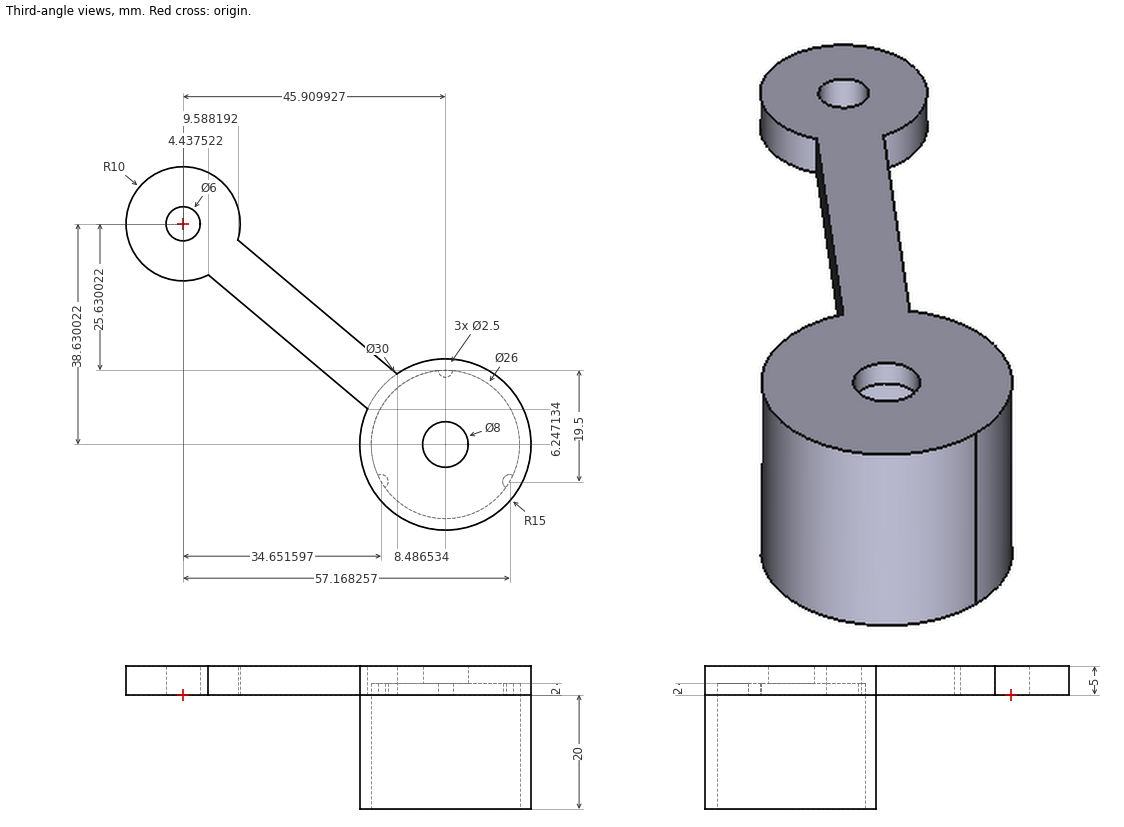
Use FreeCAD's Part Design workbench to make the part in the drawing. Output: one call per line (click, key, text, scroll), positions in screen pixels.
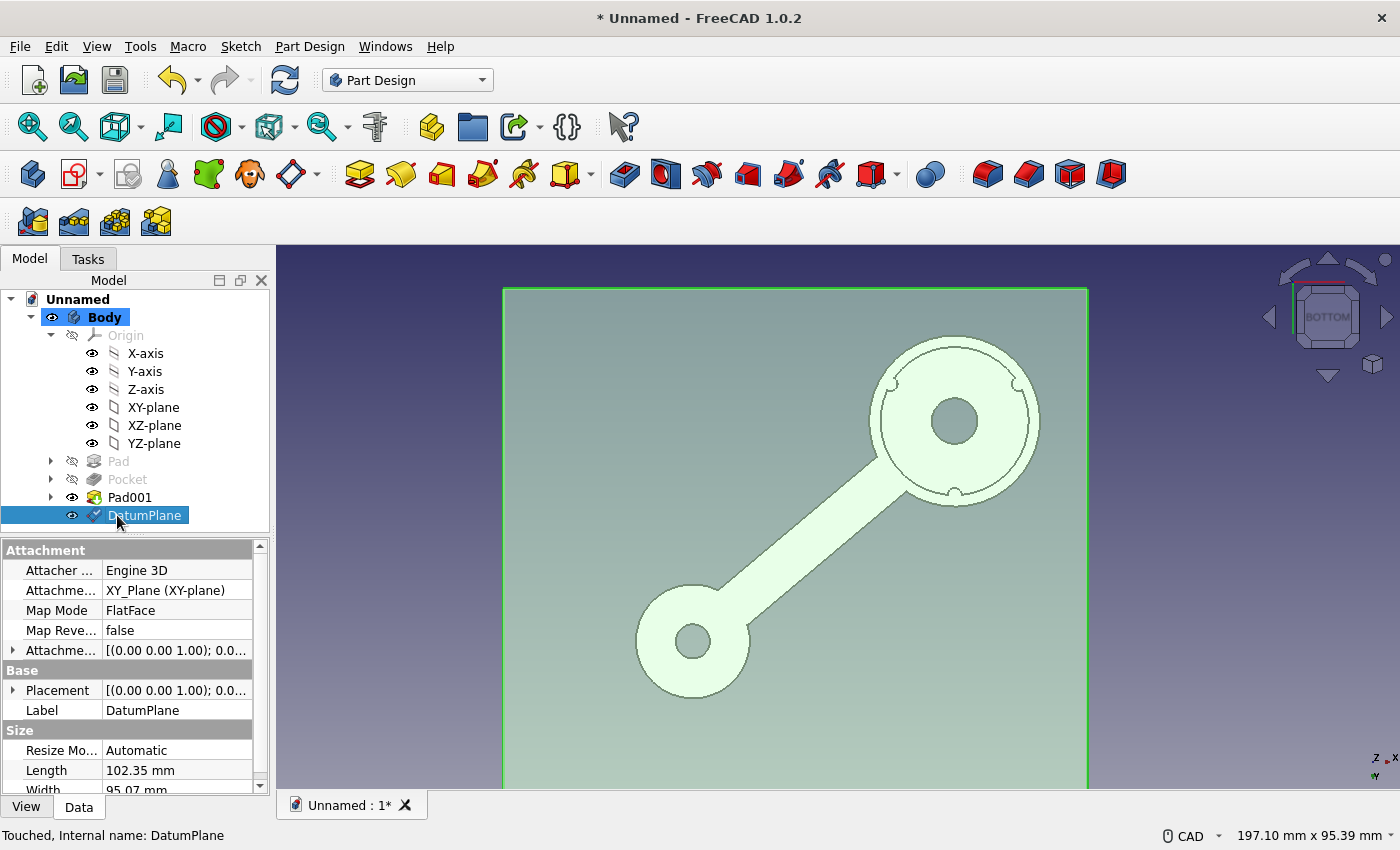
click(74, 174)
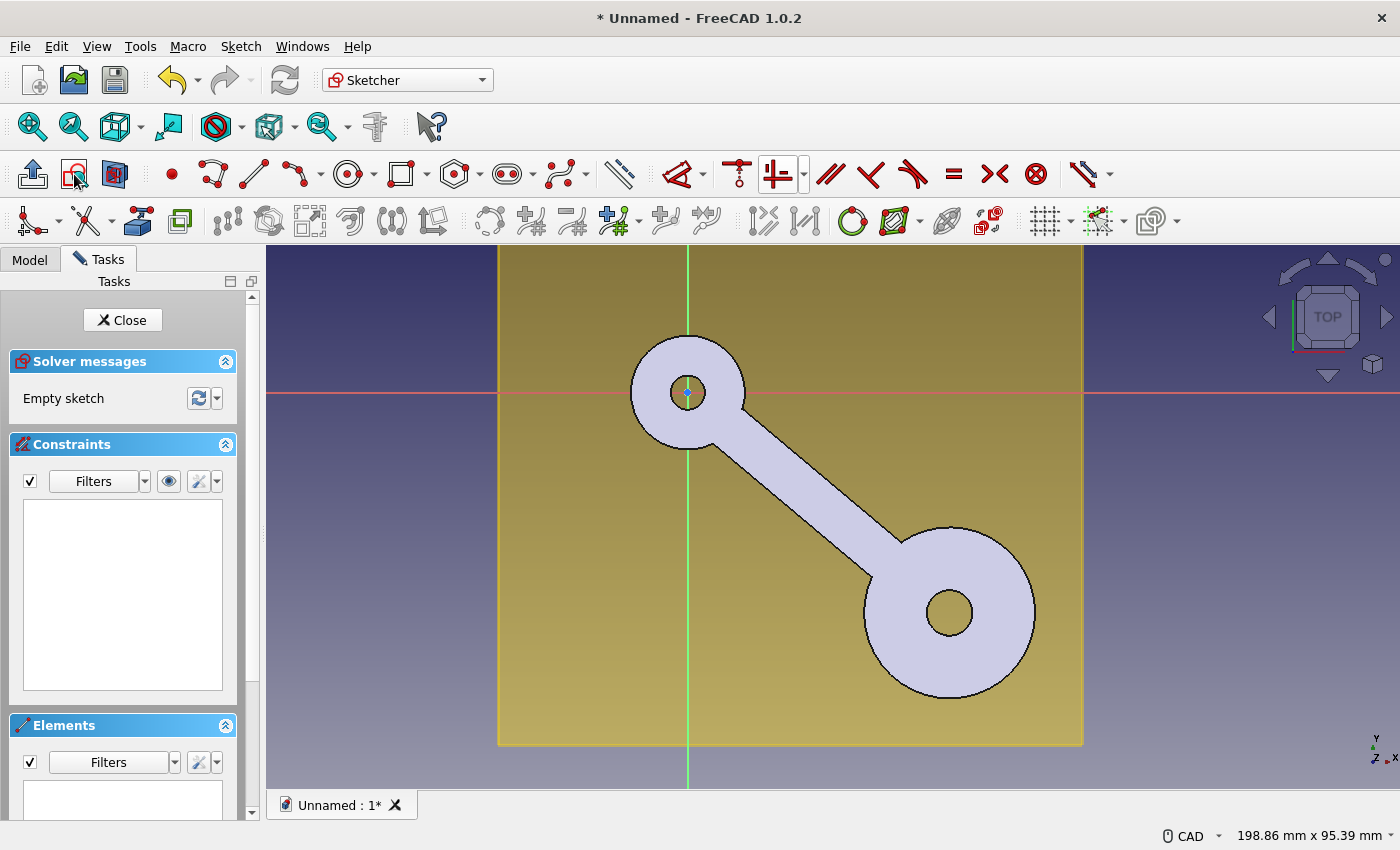
key(q)
key(s)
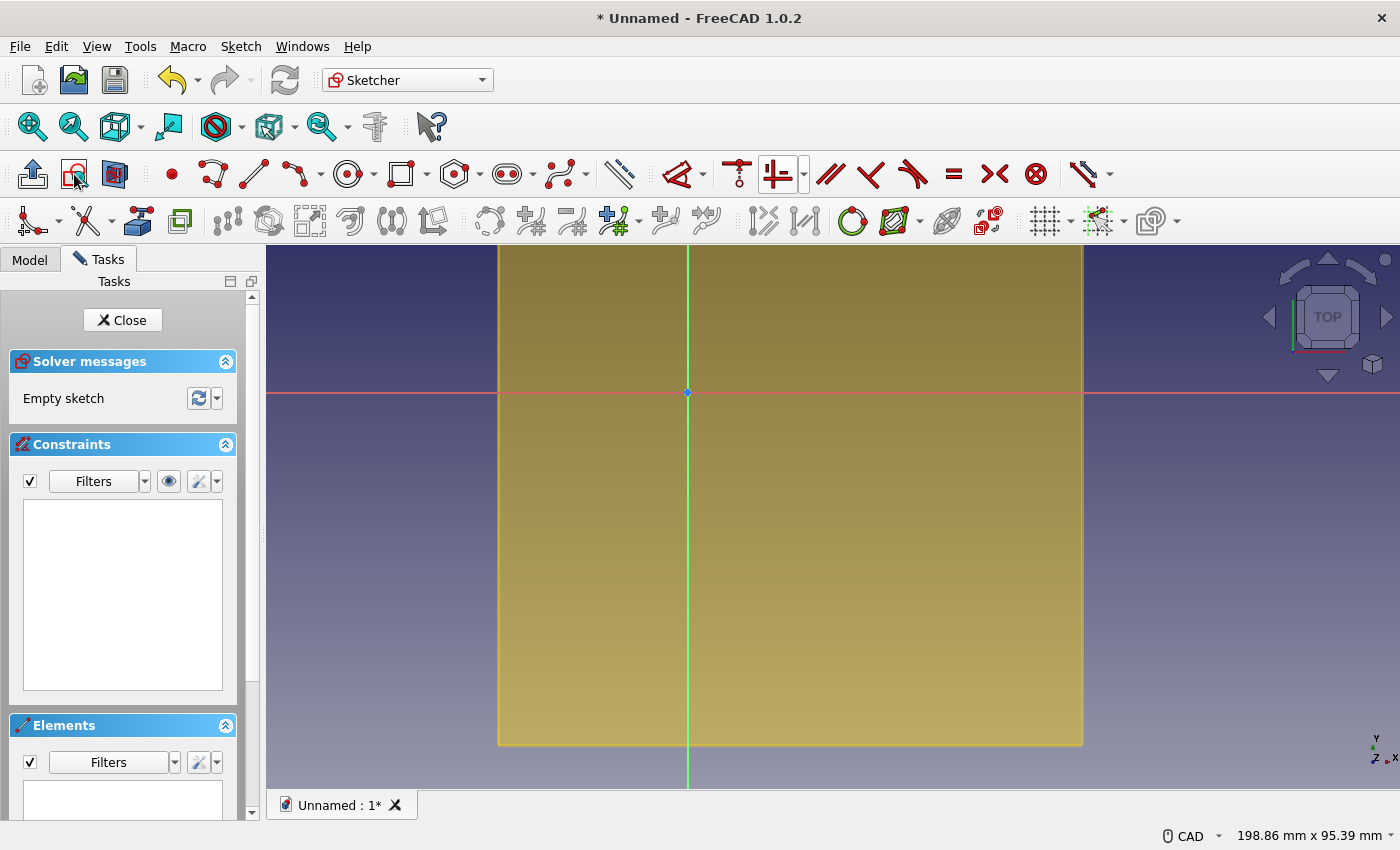
click(348, 174)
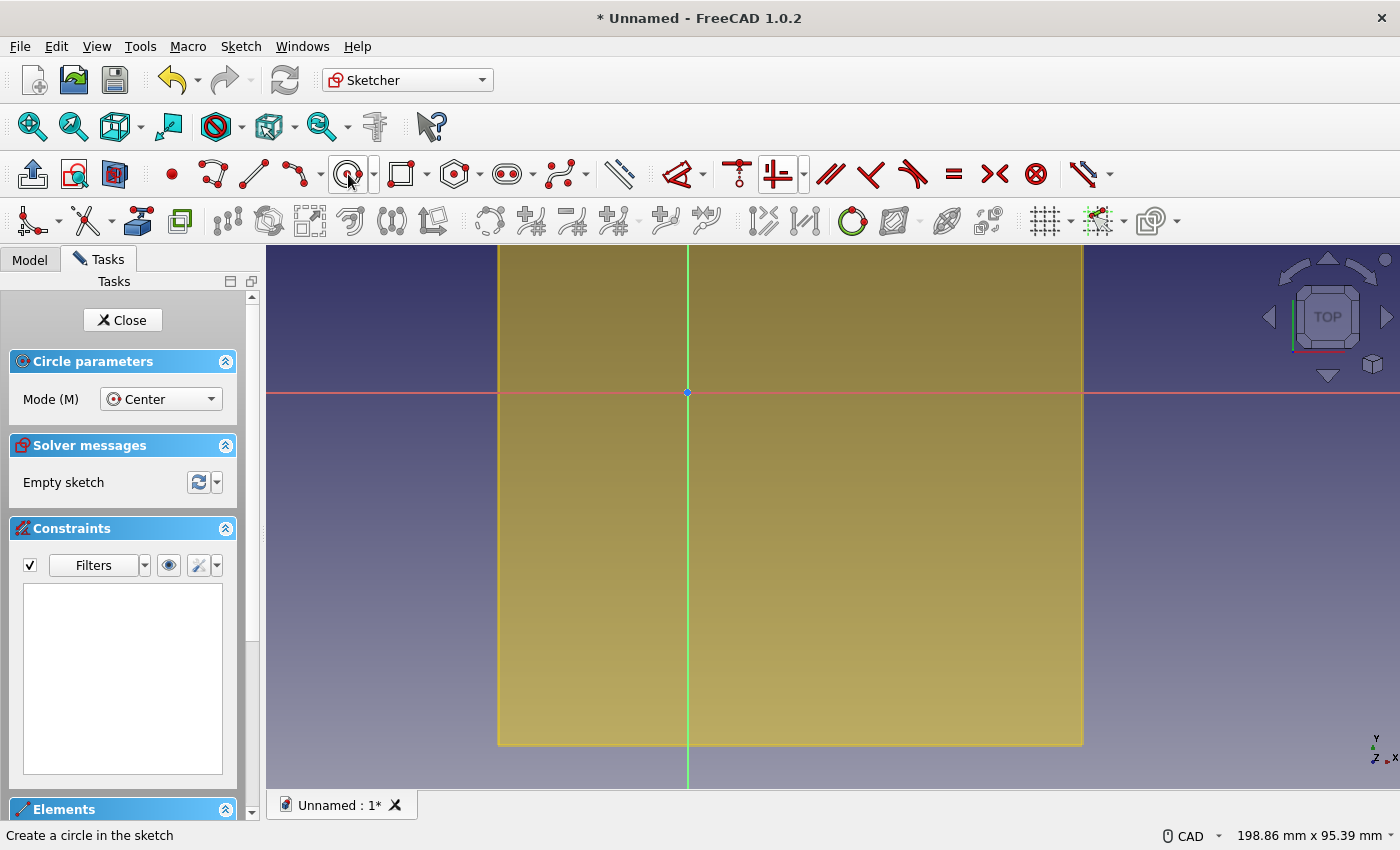
click(950, 613)
move(1010, 552)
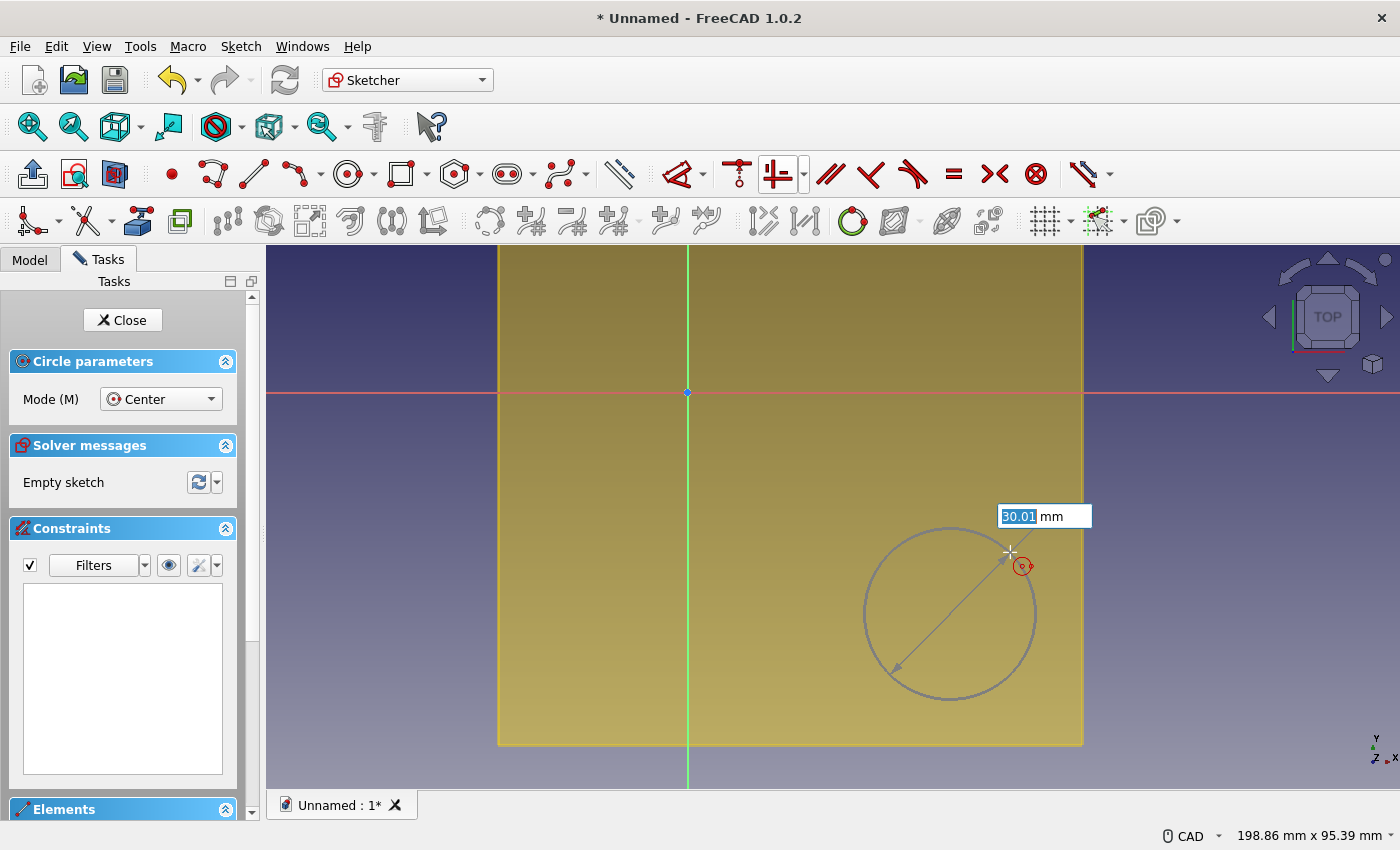
text(30)
key(Return)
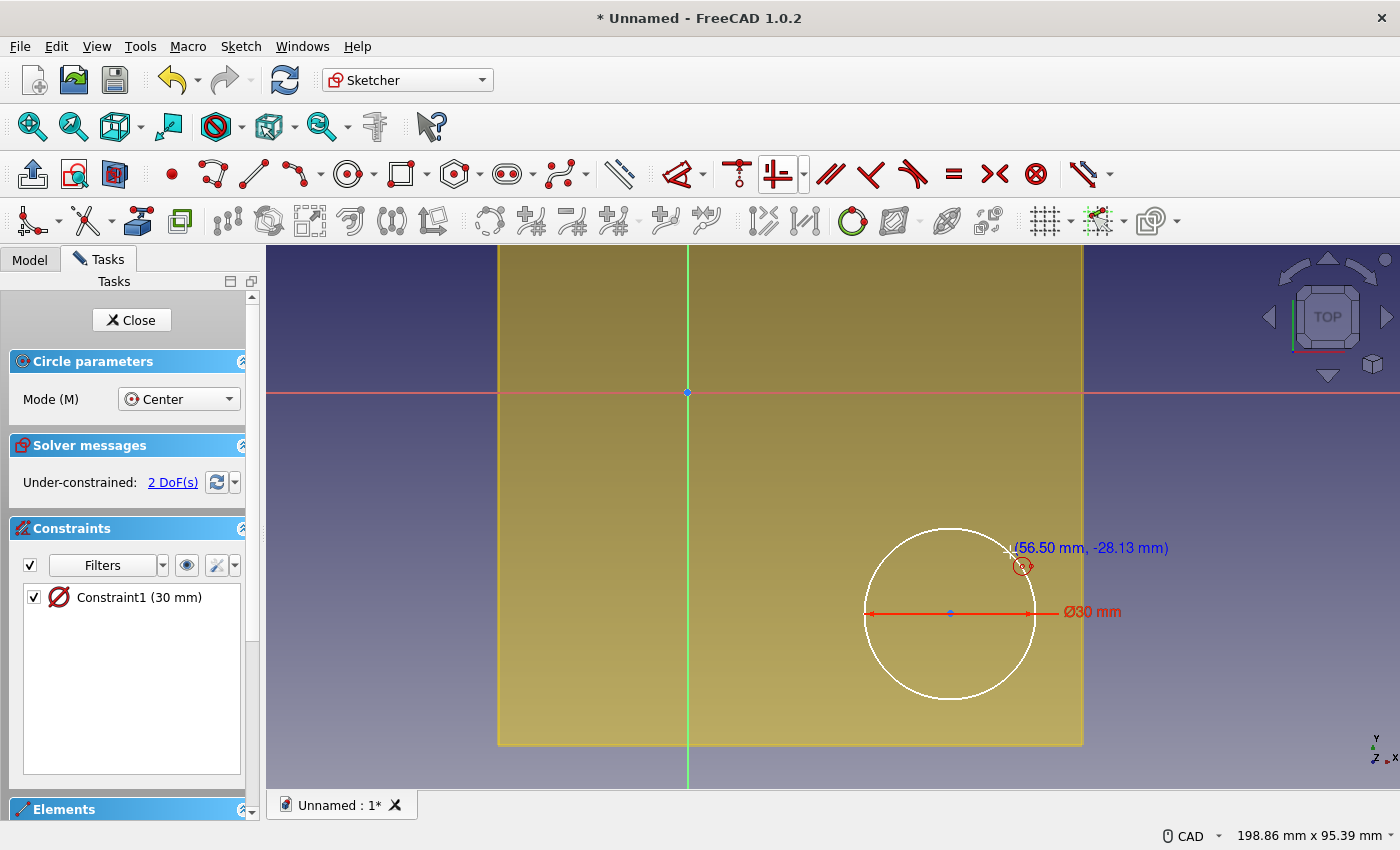
click(950, 614)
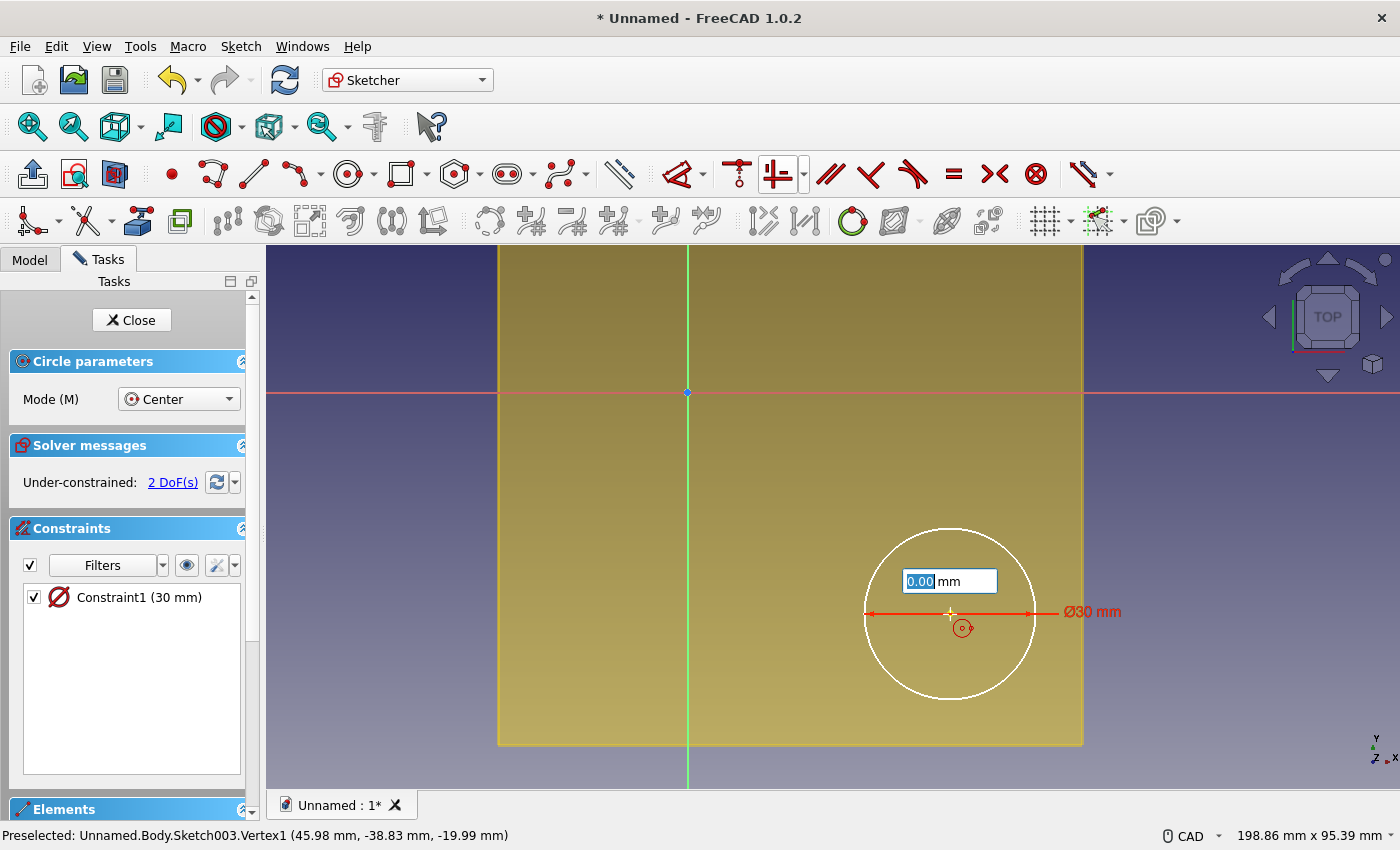
scroll(1002, 665, up, 2)
move(1002, 665)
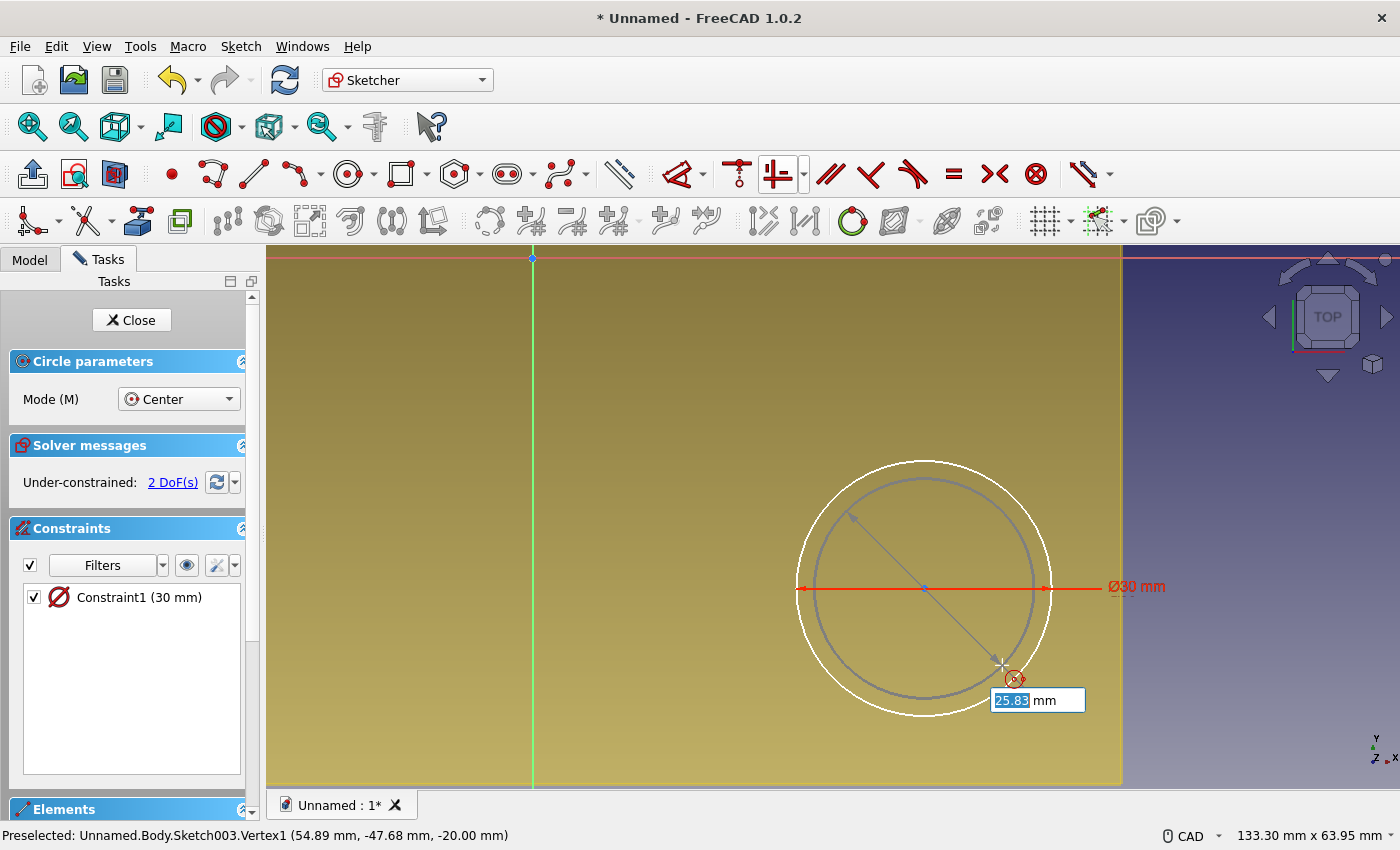
text(26)
key(Return)
key(Escape)